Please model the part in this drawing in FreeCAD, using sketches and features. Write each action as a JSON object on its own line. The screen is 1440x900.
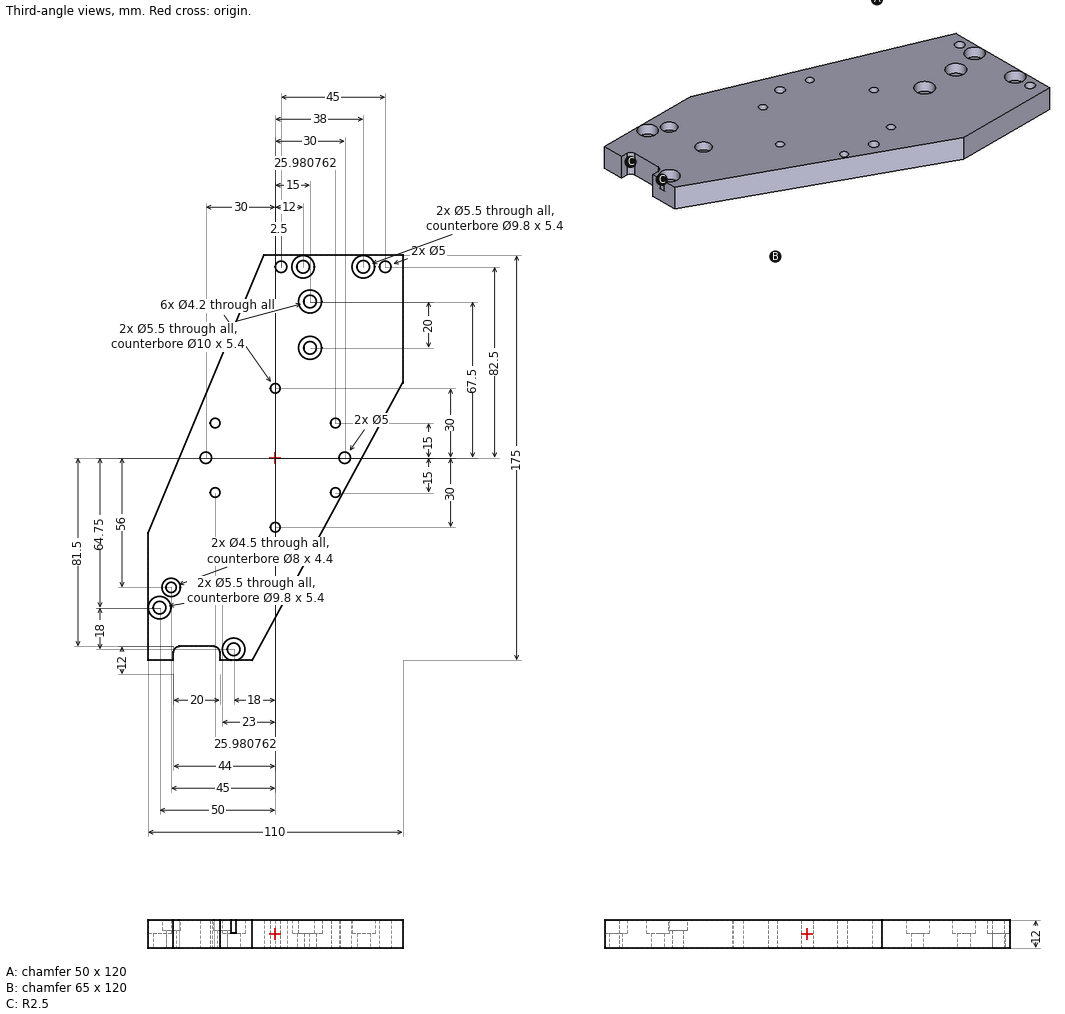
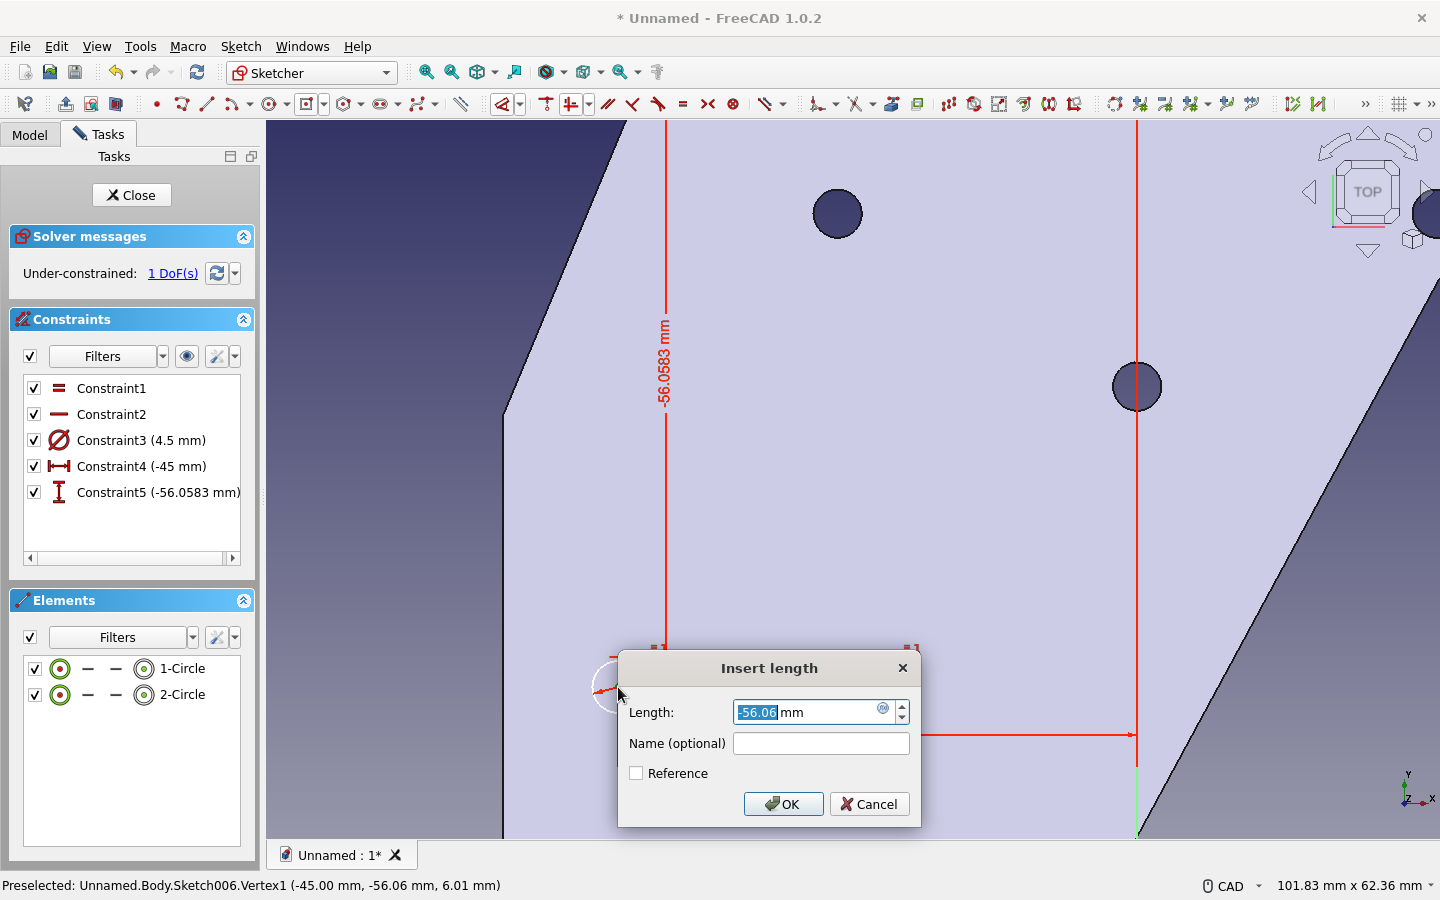
{"action": "type", "text": "-56"}
{"action": "key", "text": "Return"}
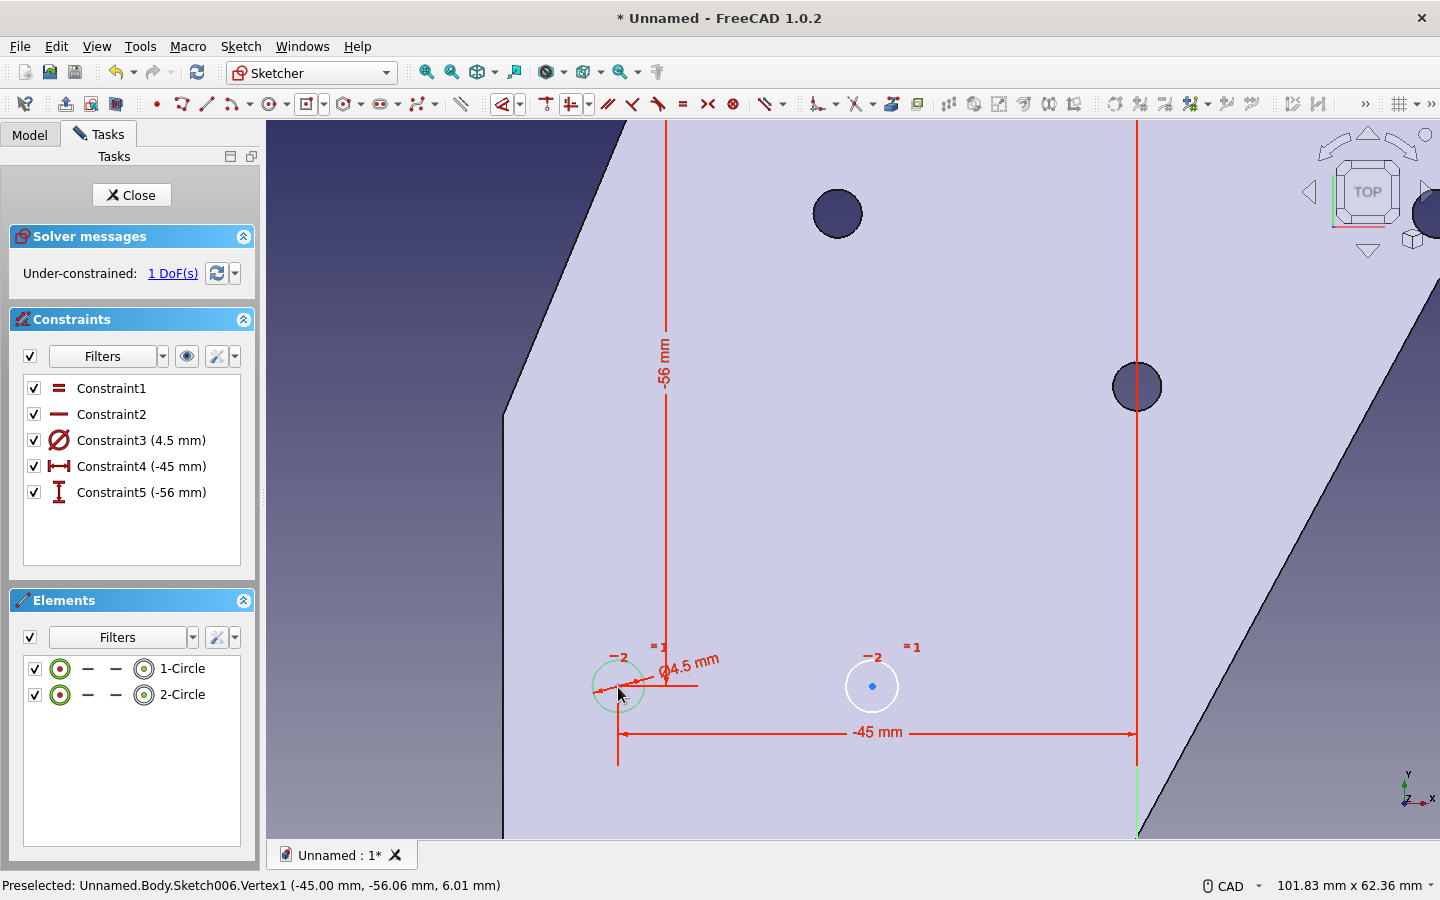
{"action": "left_click", "coordinate": [872, 686]}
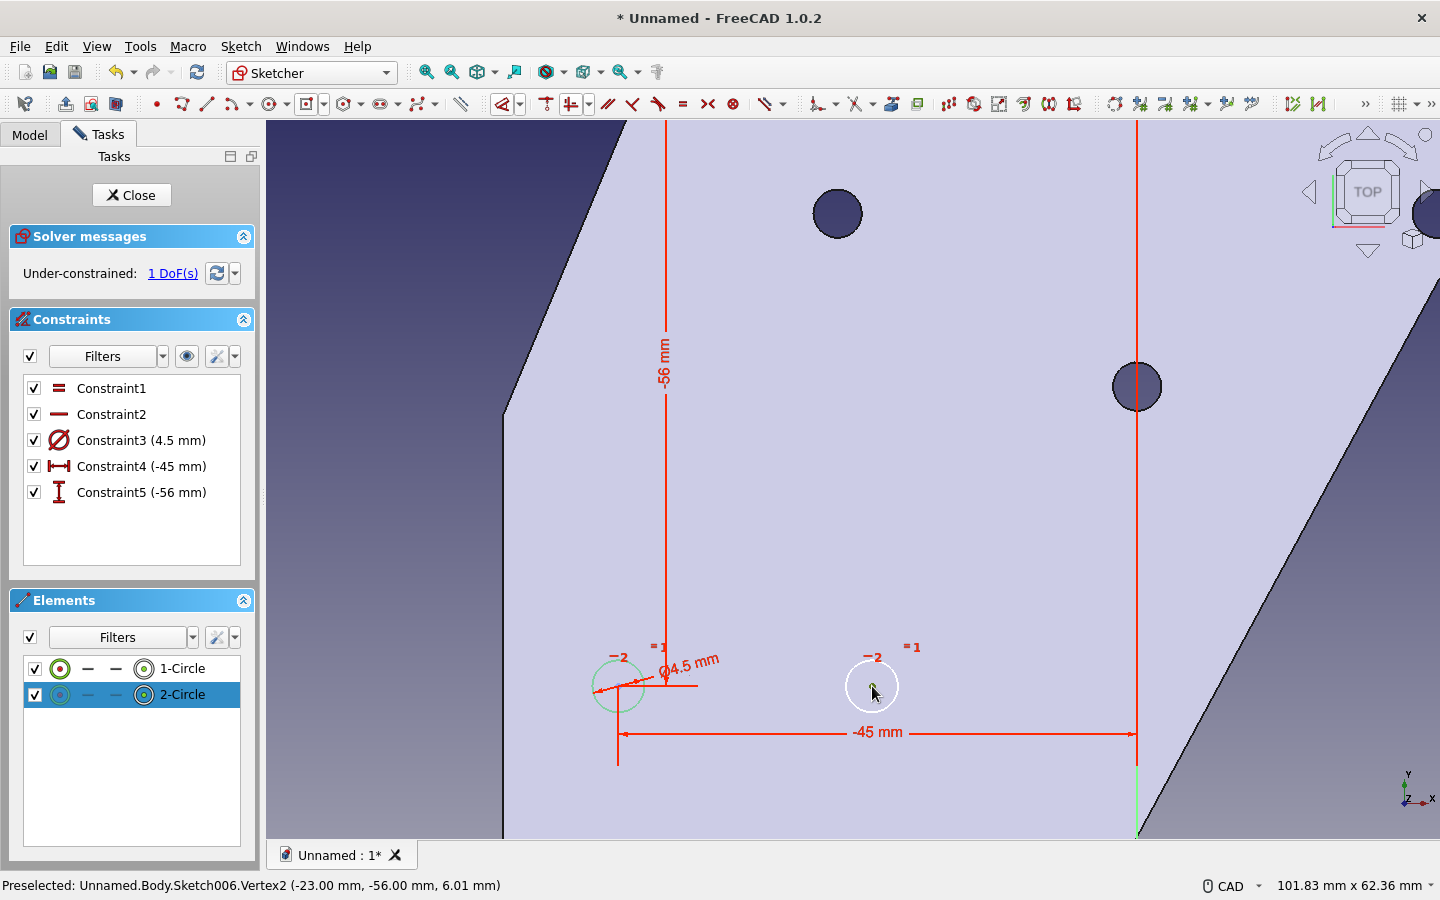
{"action": "key", "text": "l"}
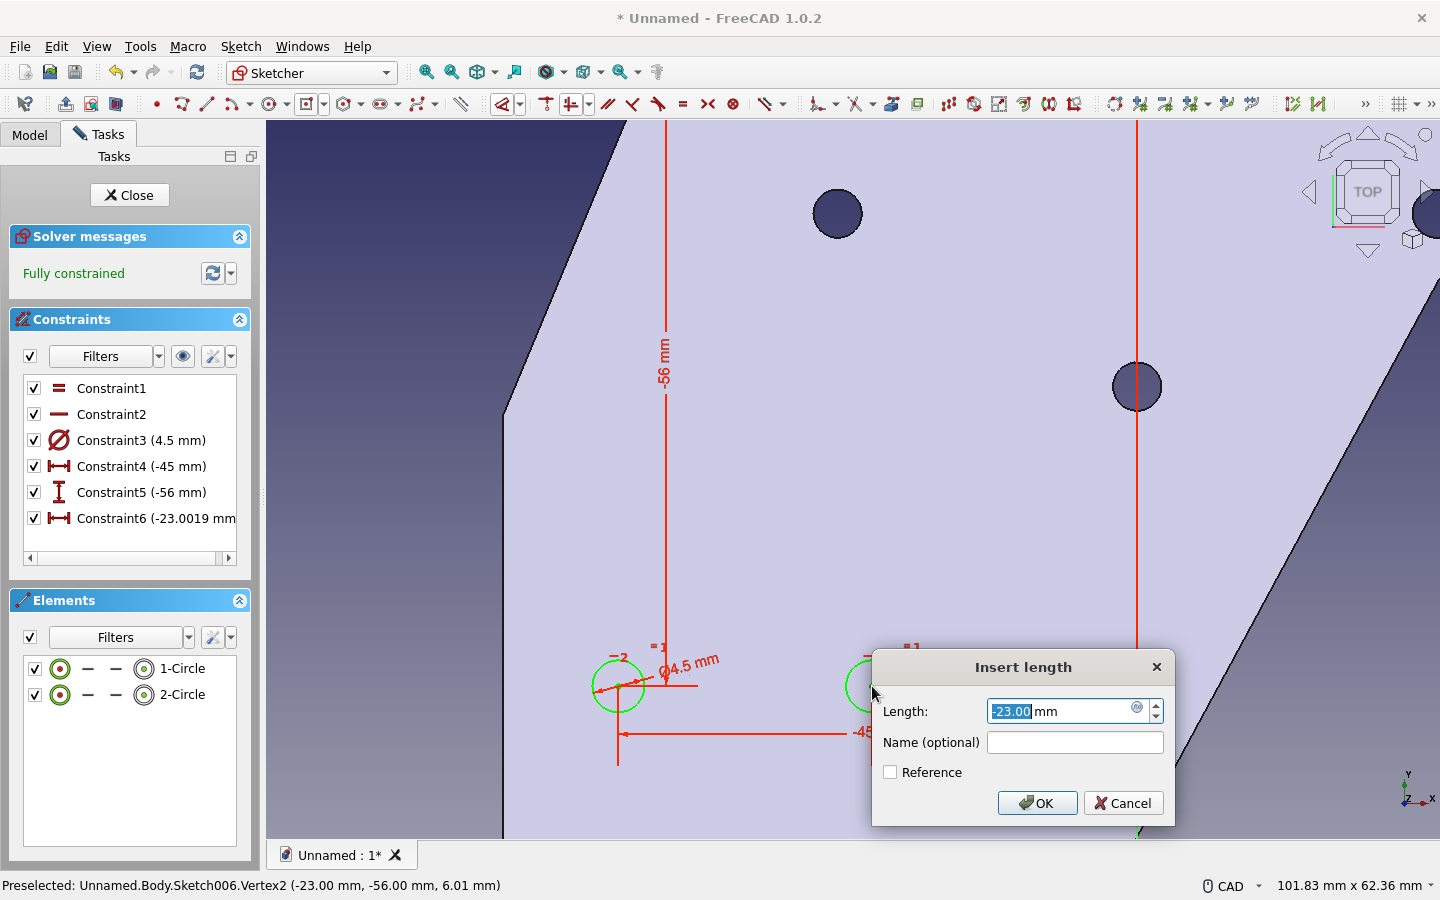
{"action": "type", "text": "-23"}
{"action": "key", "text": "Return"}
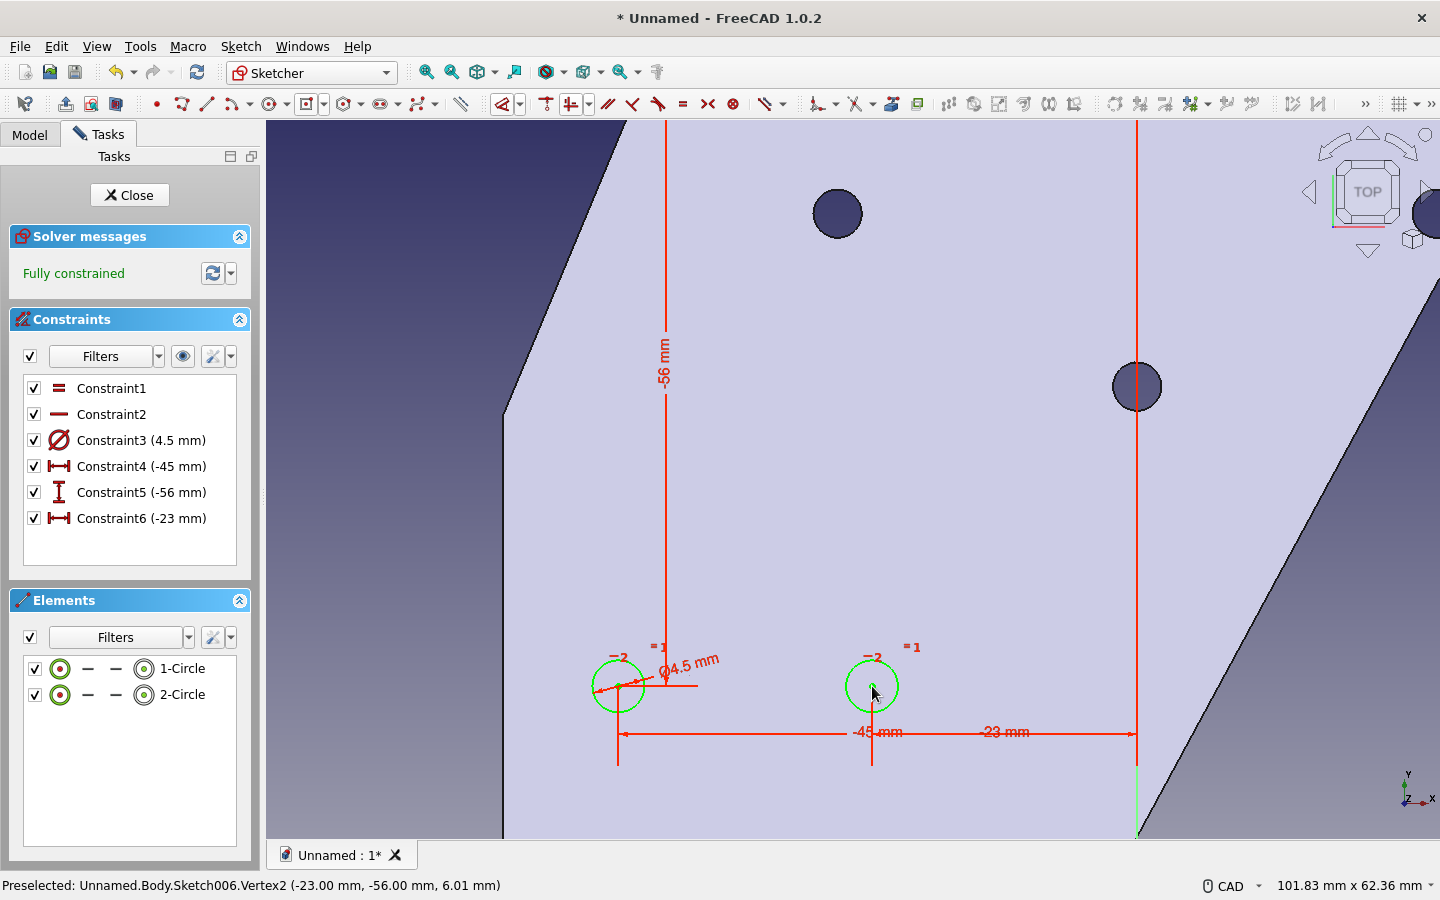
{"action": "left_click", "coordinate": [130, 195]}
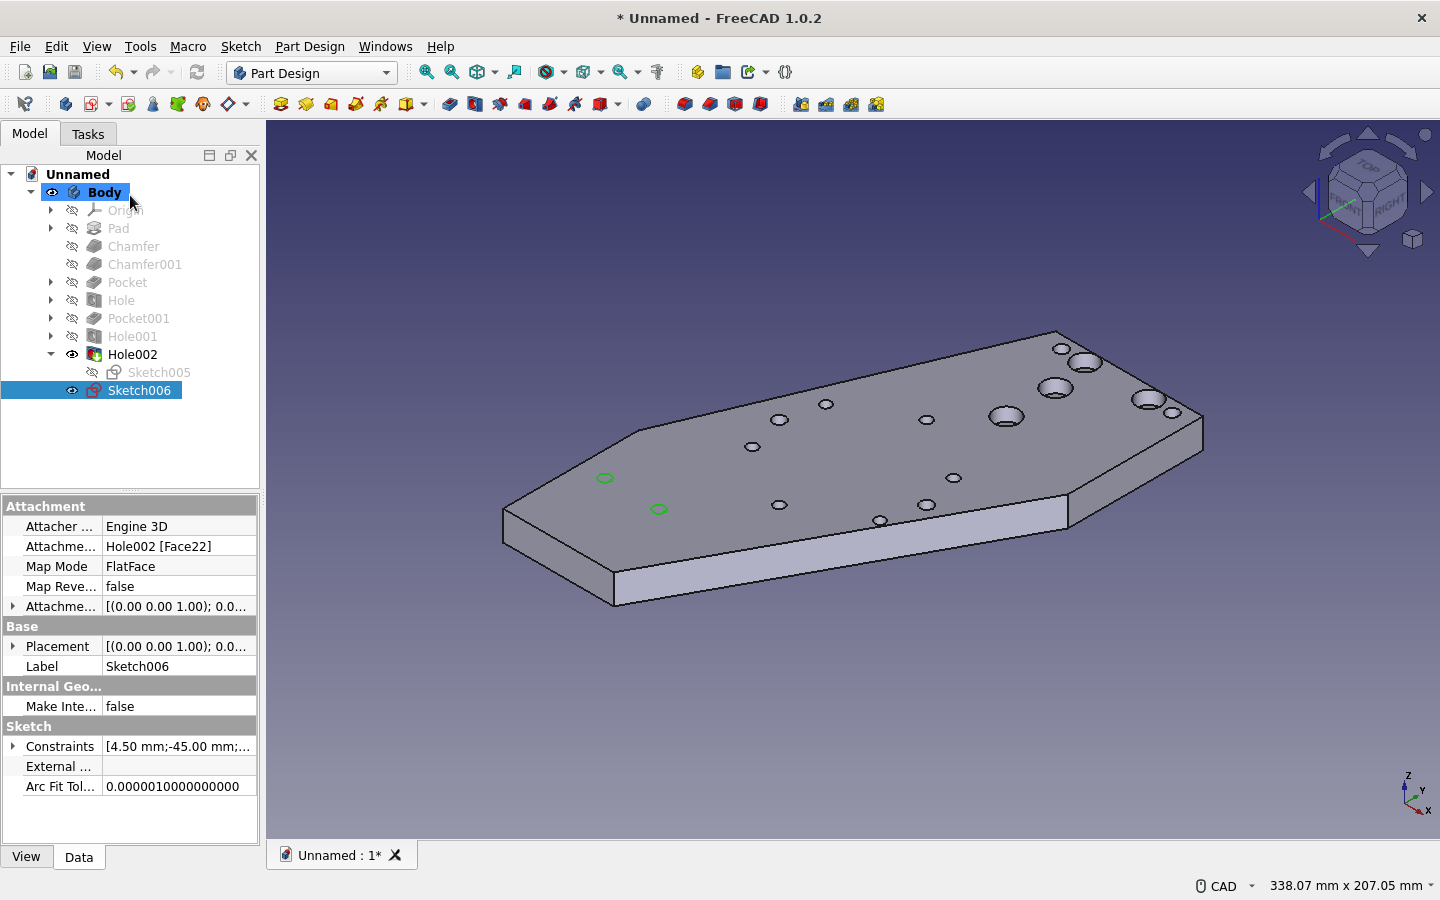
{"action": "left_click", "coordinate": [475, 104]}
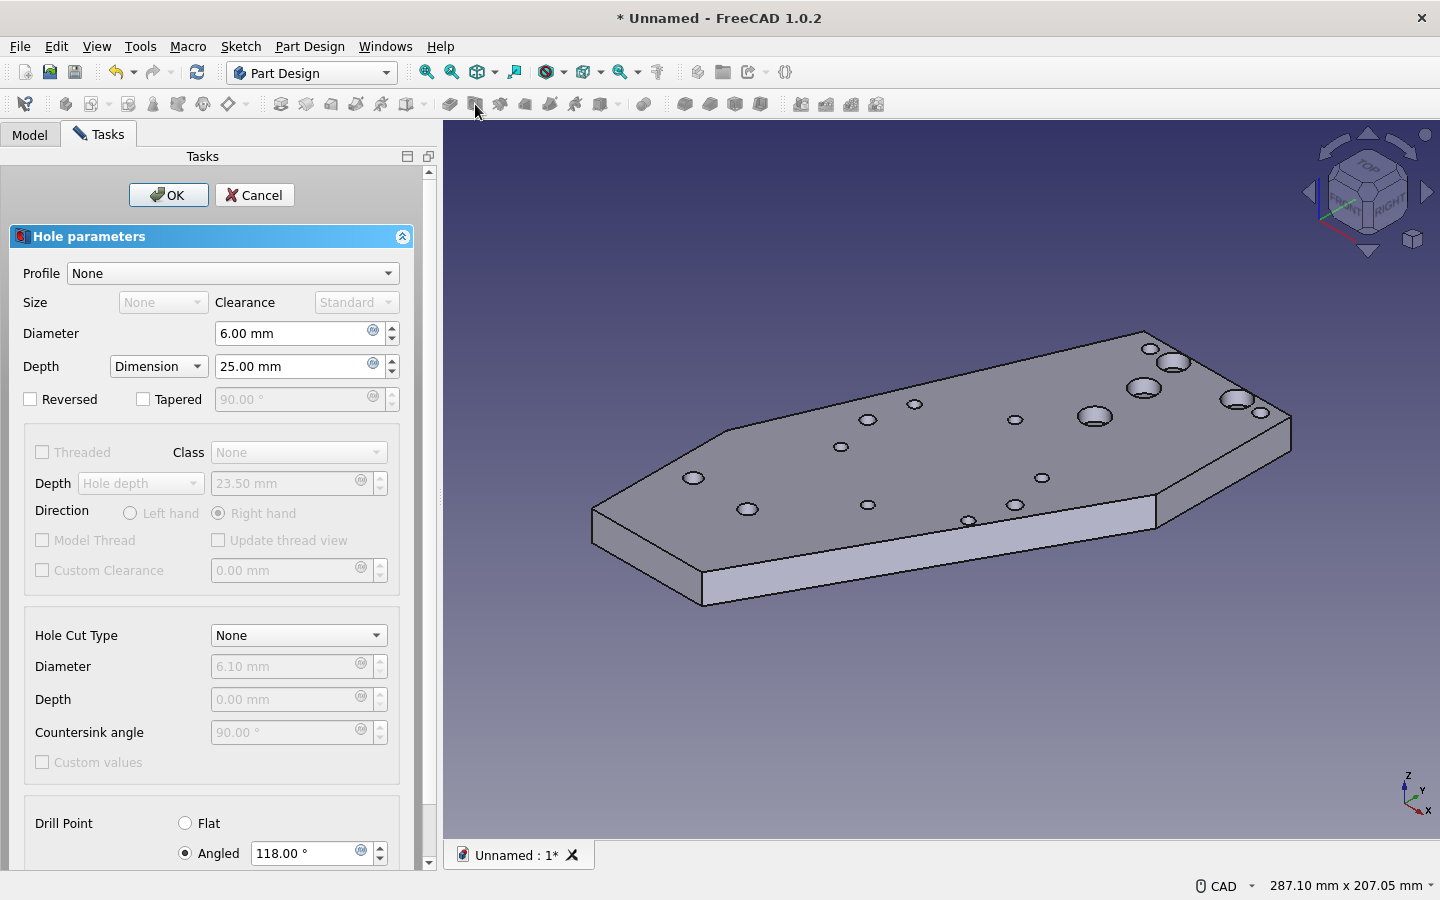
{"action": "triple_click", "coordinate": [300, 334]}